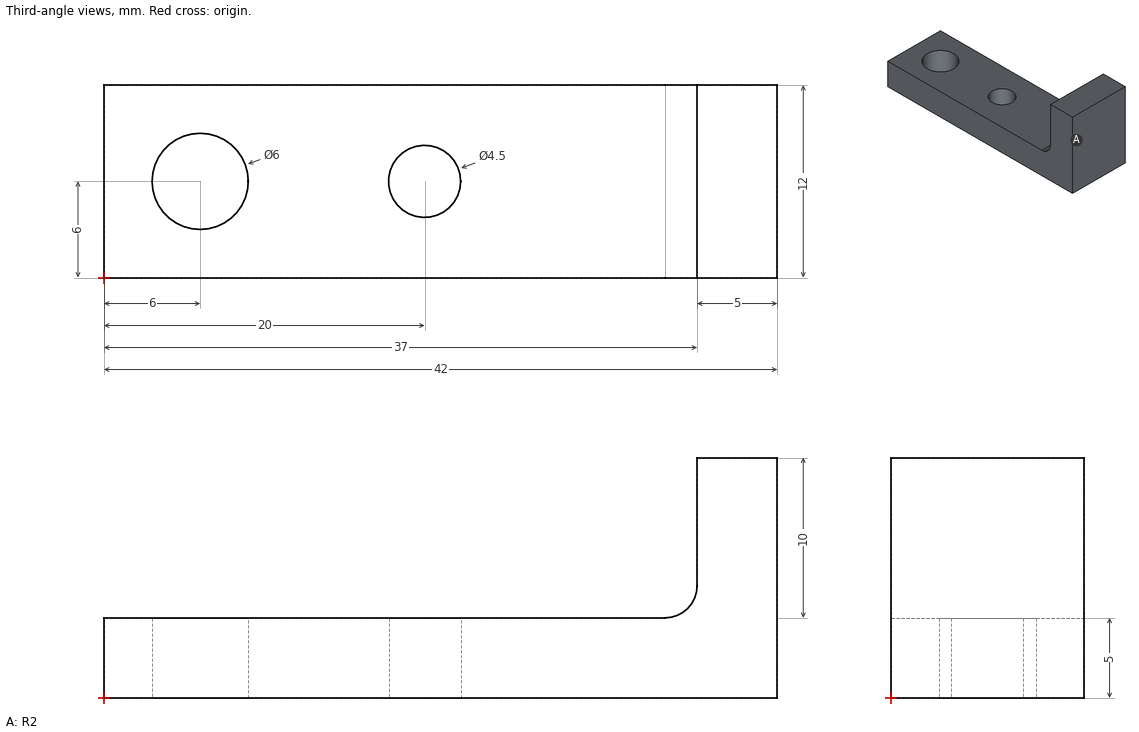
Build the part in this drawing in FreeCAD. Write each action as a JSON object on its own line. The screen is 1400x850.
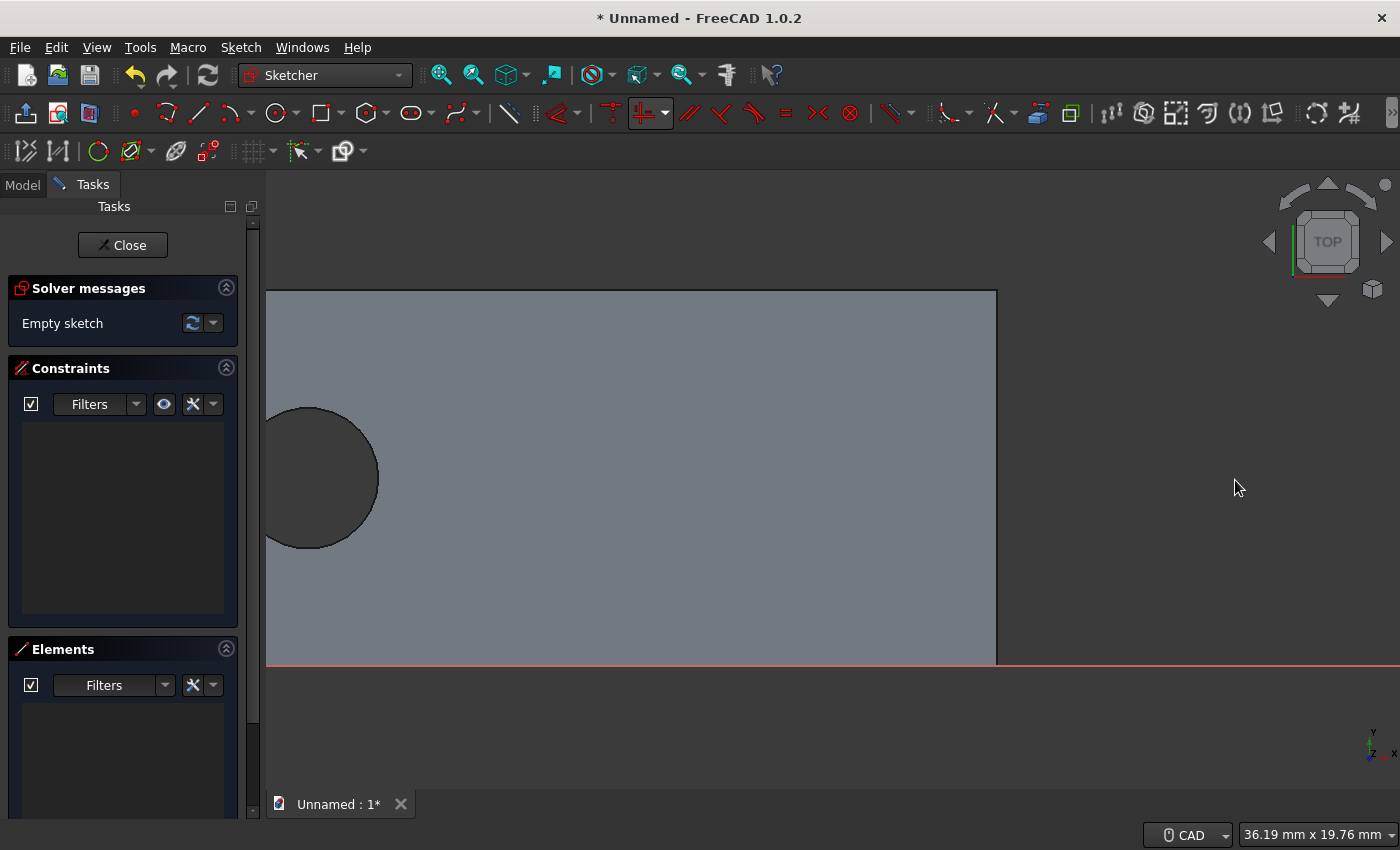
{"action": "key", "text": "g r"}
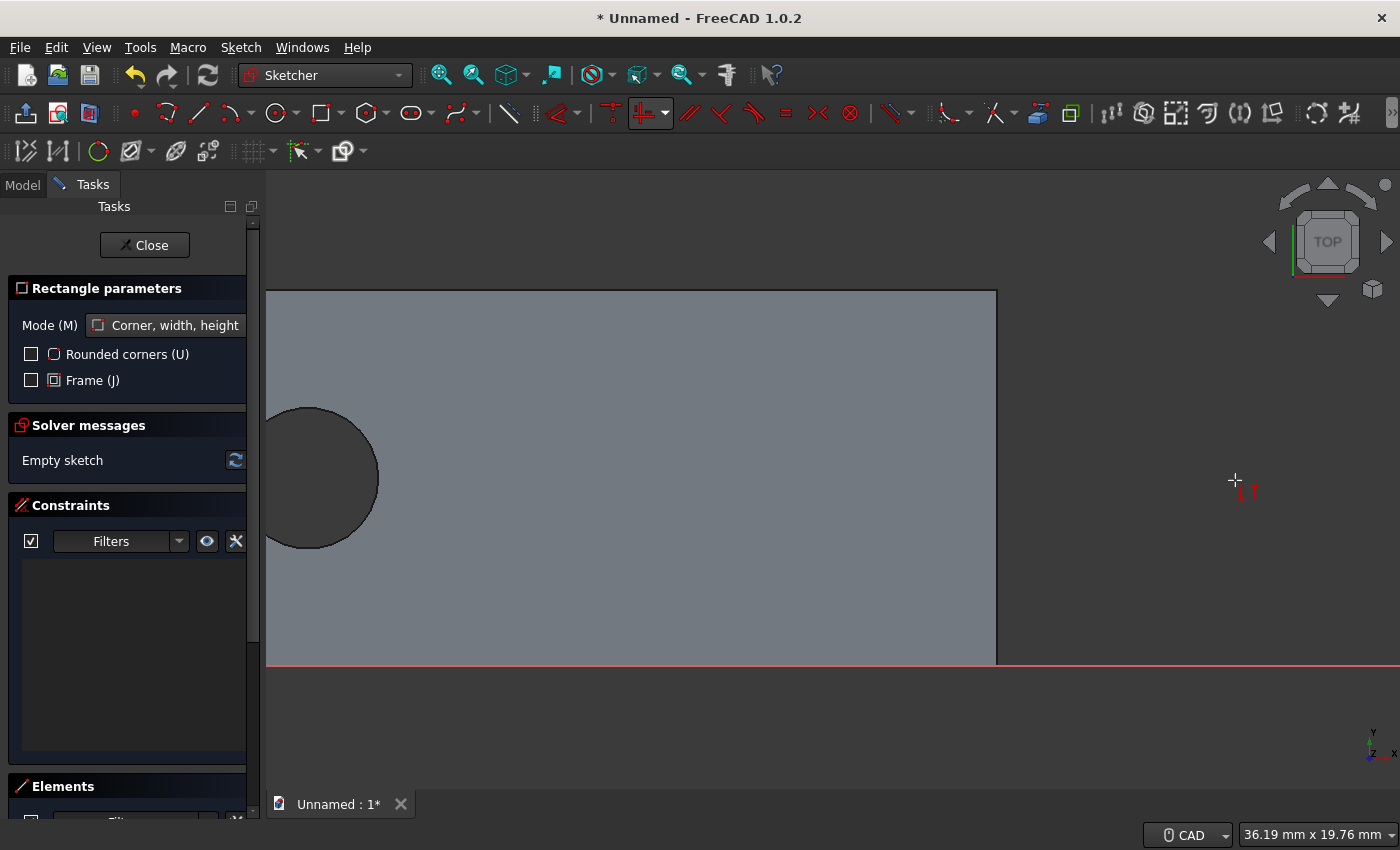
{"action": "left_click", "coordinate": [841, 290]}
{"action": "left_click", "coordinate": [997, 666]}
{"action": "key", "text": "Escape"}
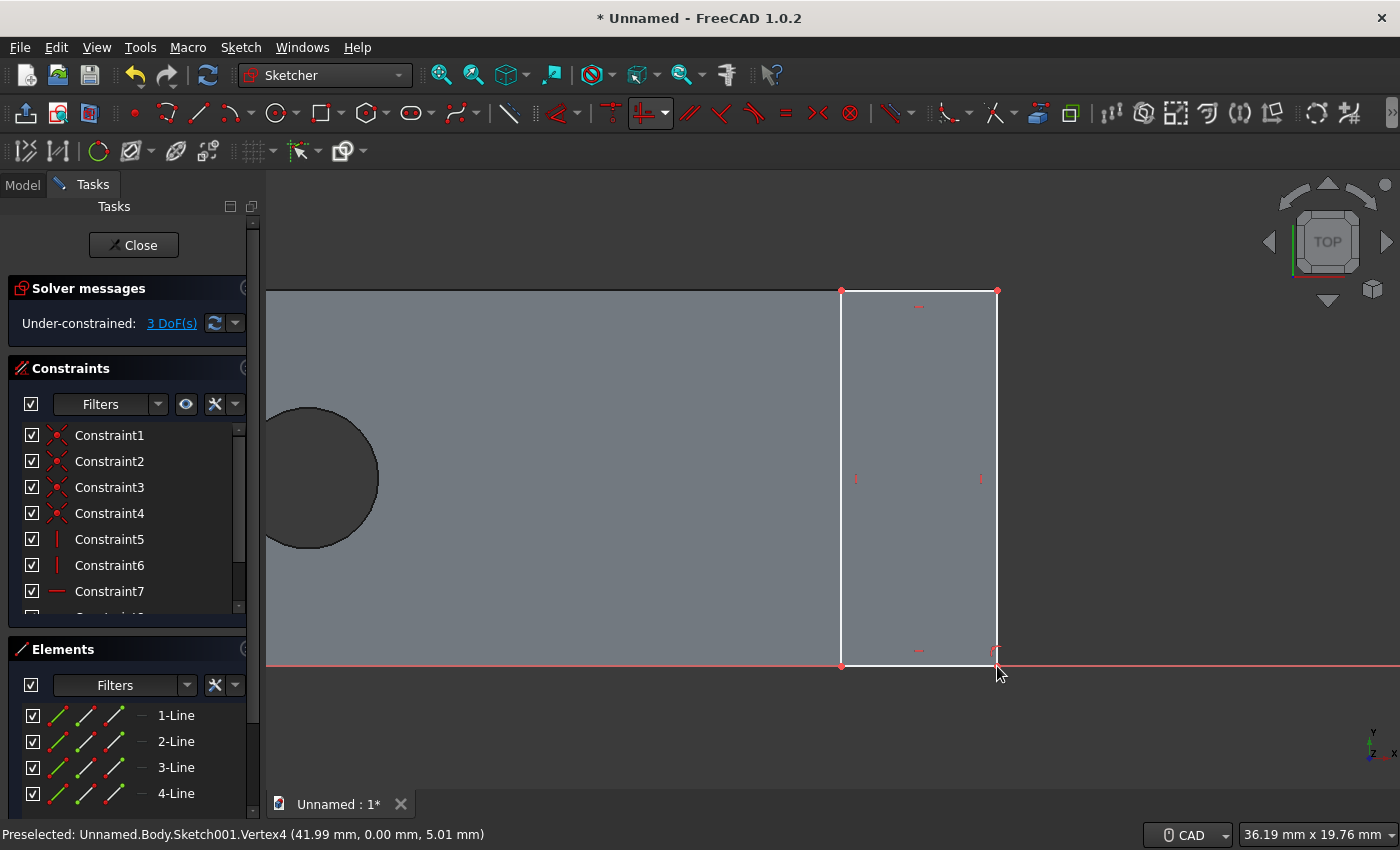
{"action": "left_click", "coordinate": [556, 114]}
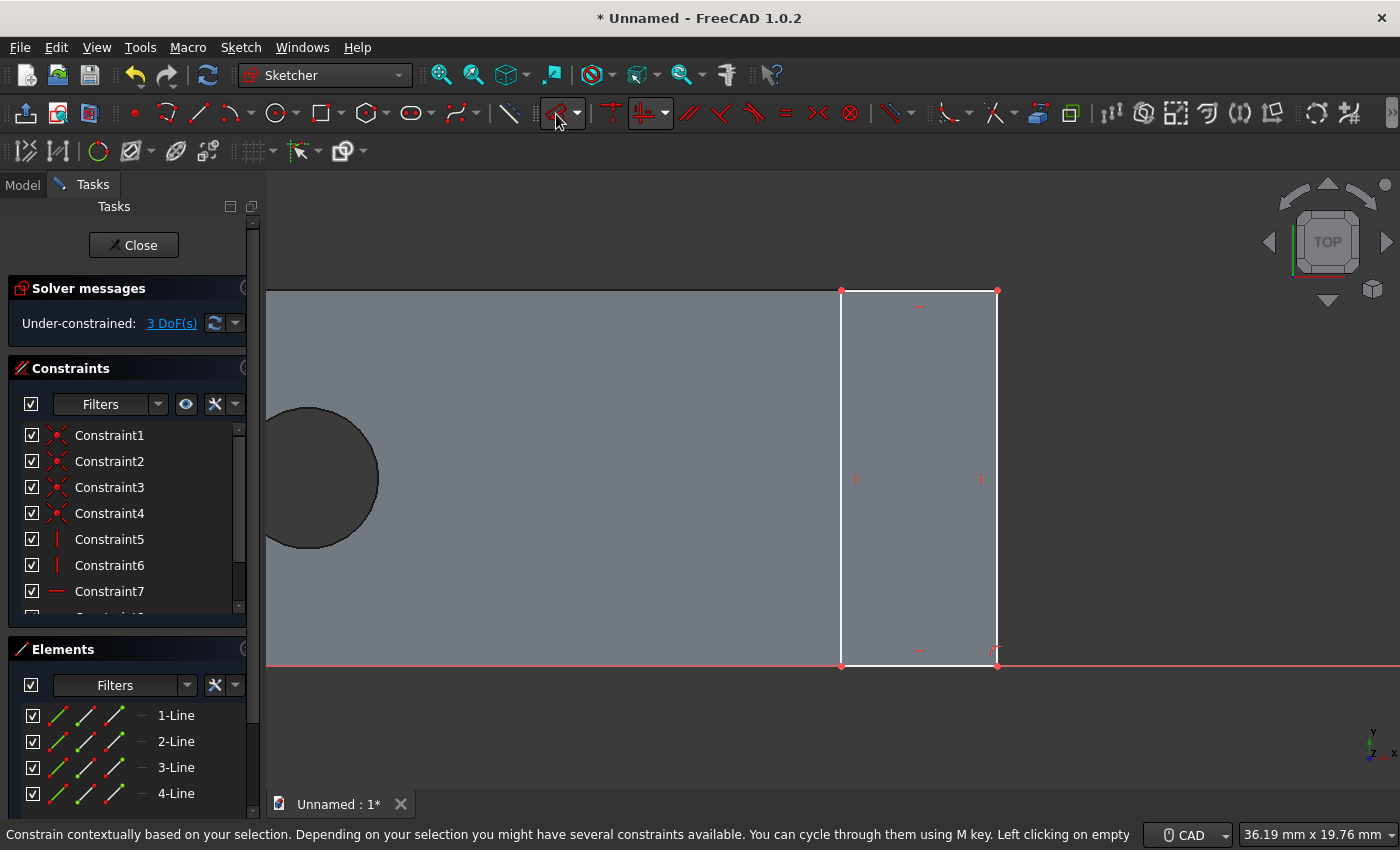
{"action": "left_click", "coordinate": [888, 666]}
{"action": "left_click", "coordinate": [919, 700]}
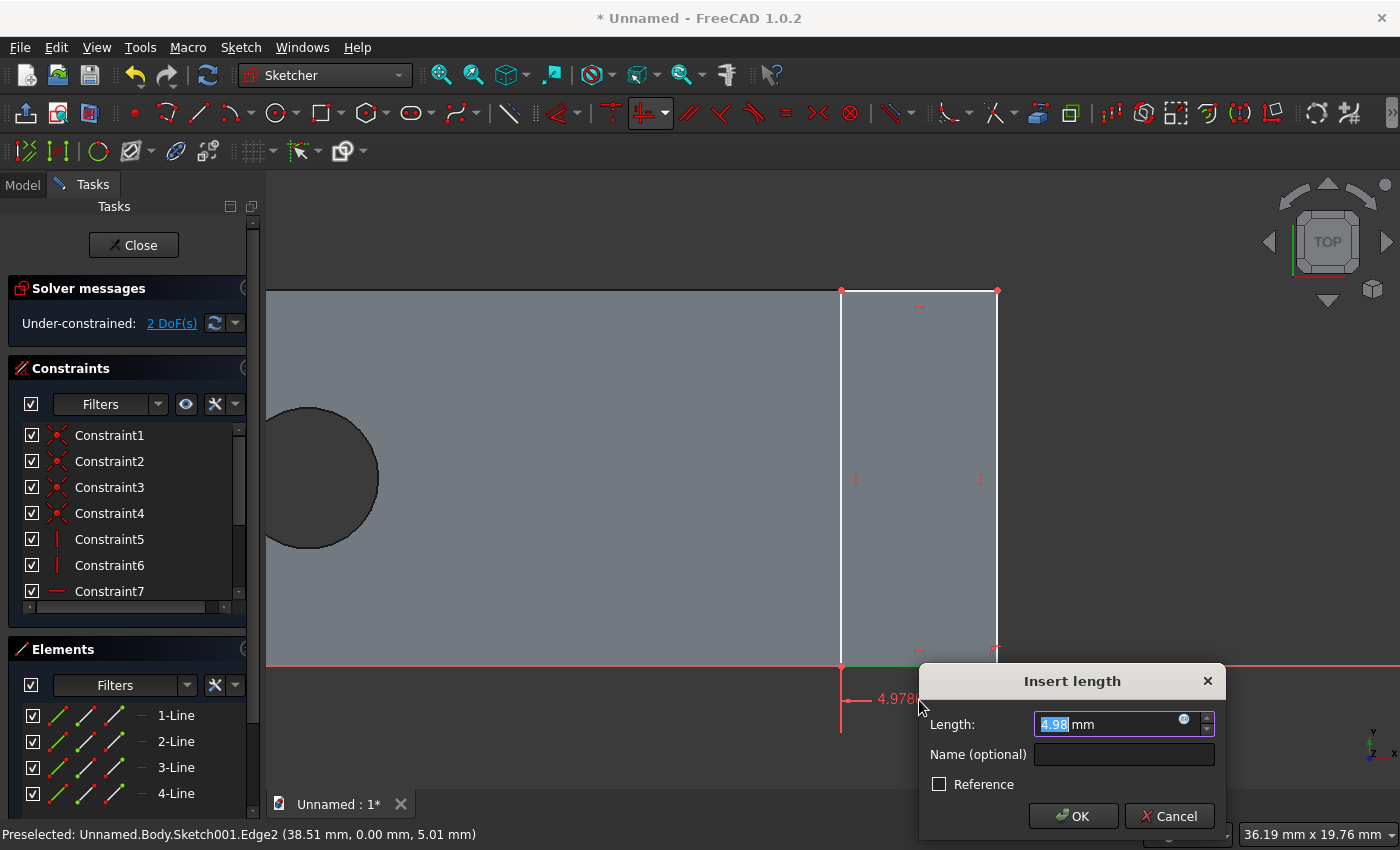
{"action": "type", "text": "5"}
{"action": "key", "text": "Return"}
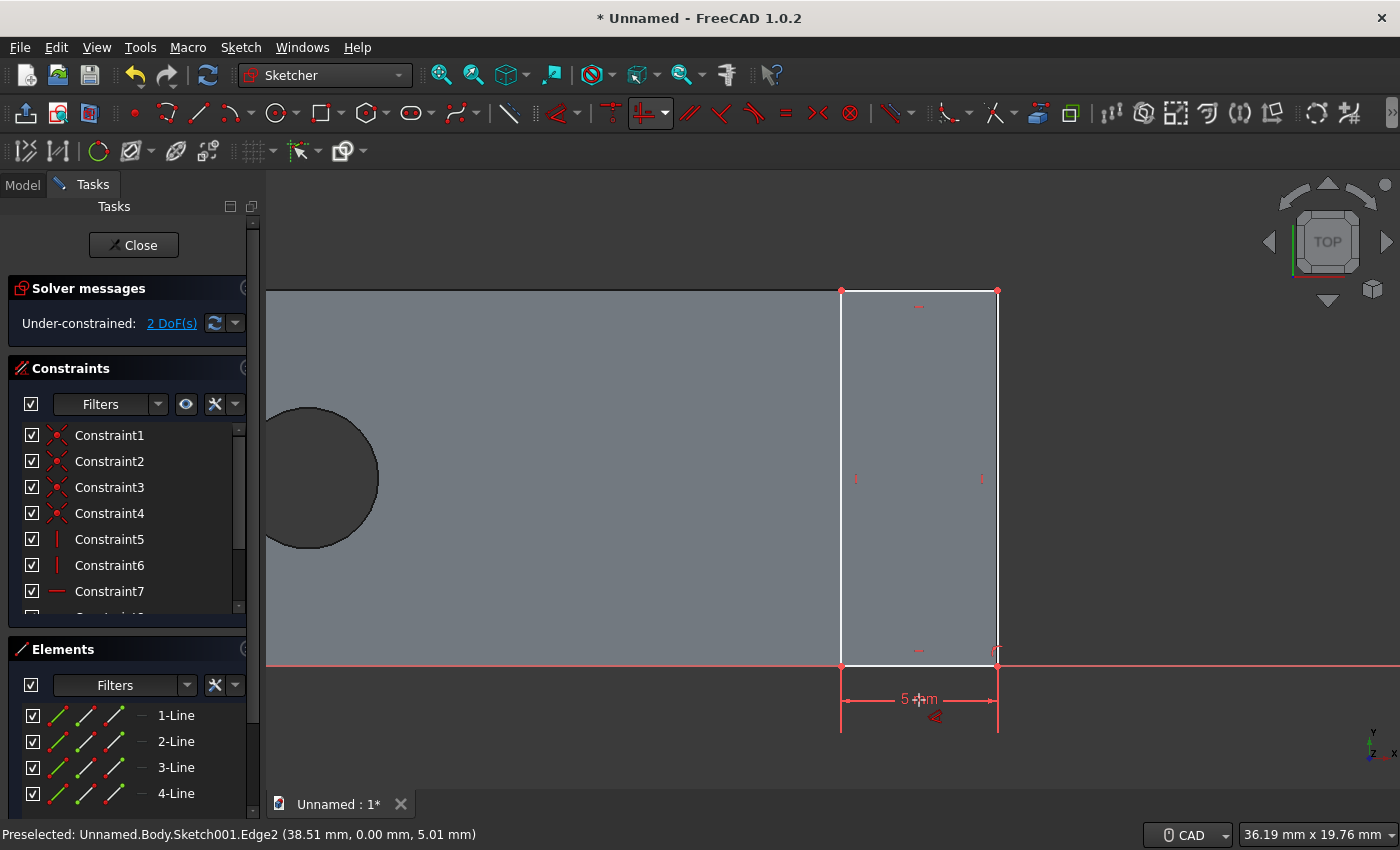
{"action": "left_click", "coordinate": [841, 404]}
{"action": "left_click", "coordinate": [807, 479]}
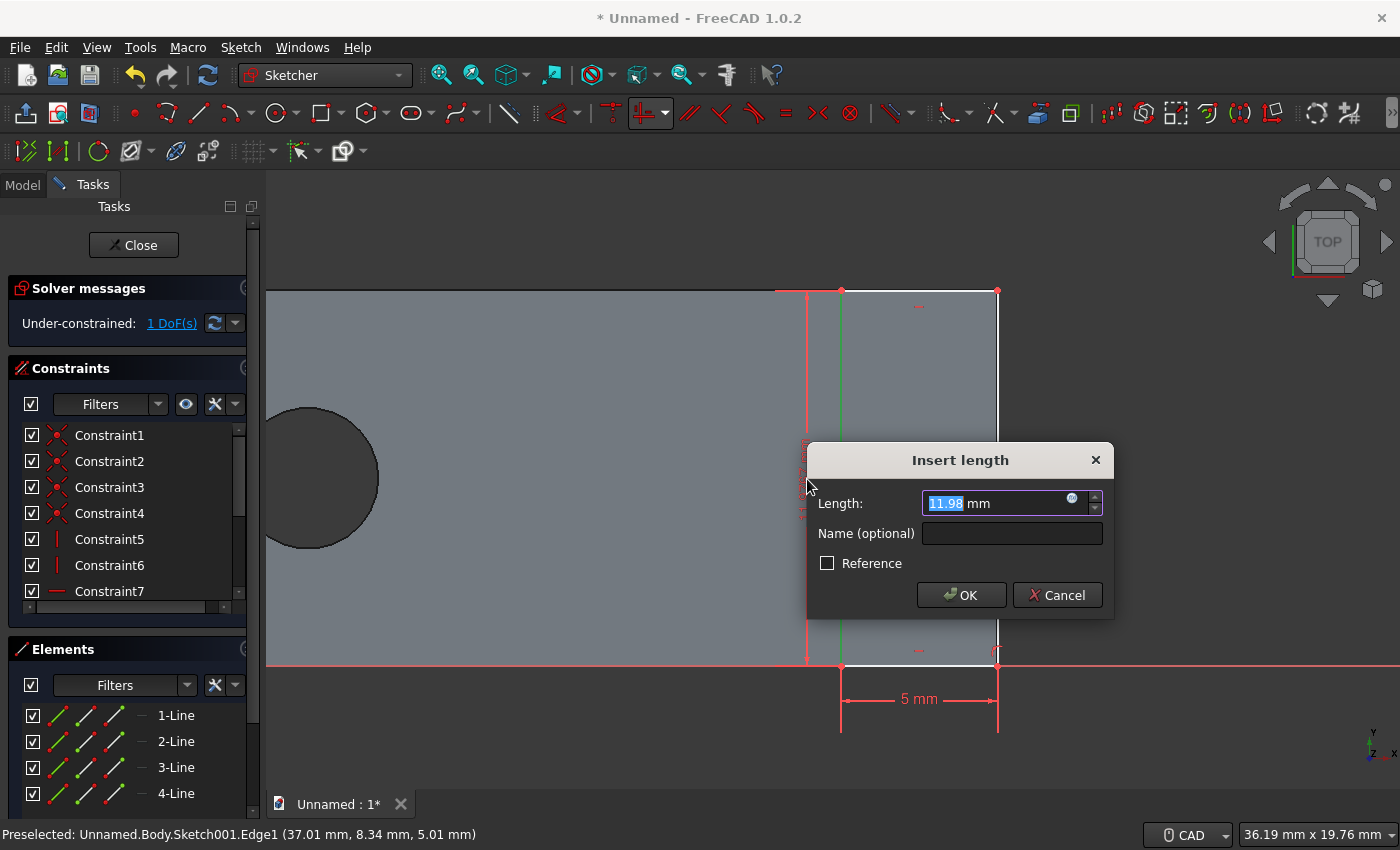
{"action": "type", "text": "12"}
{"action": "key", "text": "Return"}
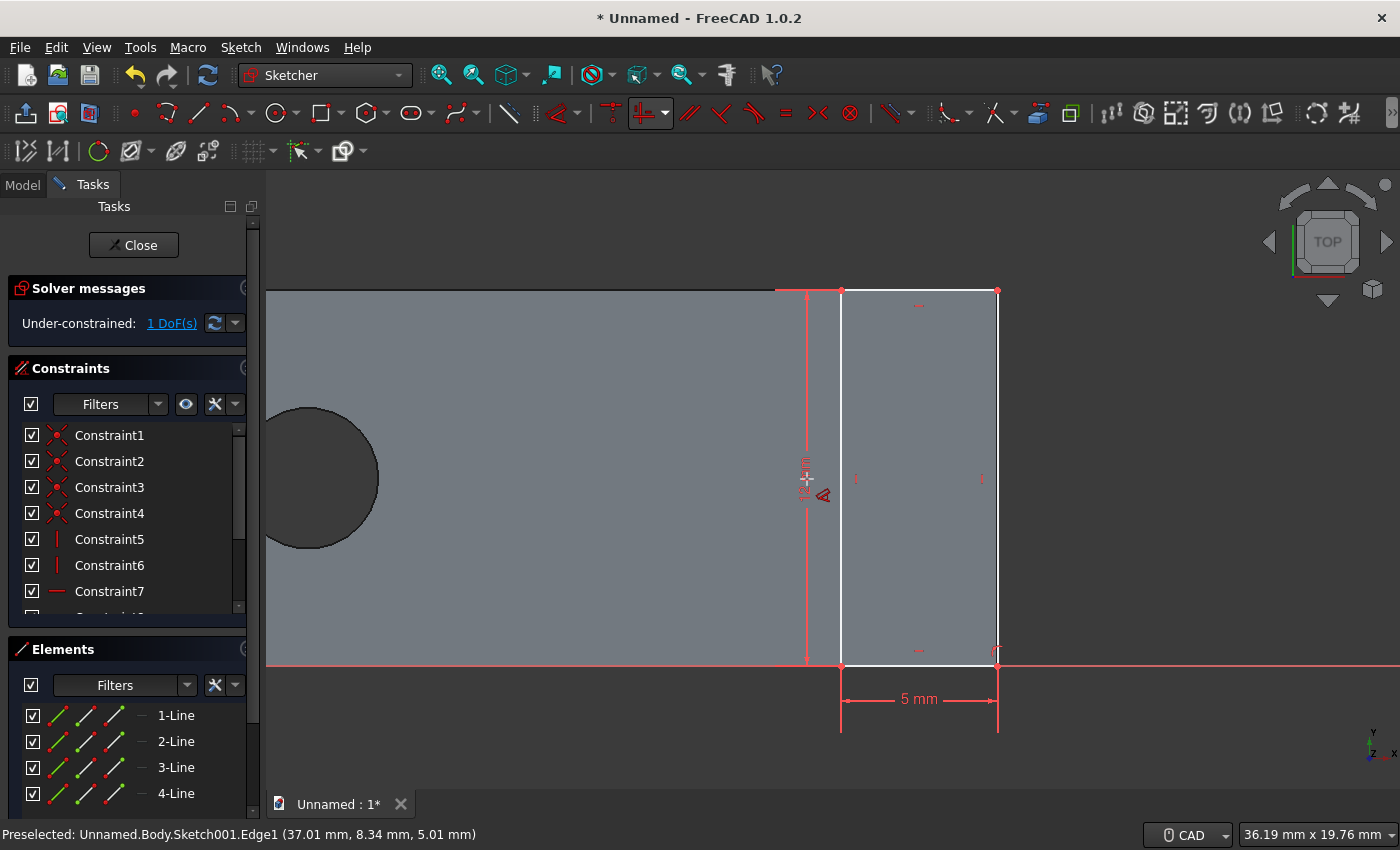
{"action": "left_click", "coordinate": [841, 290]}
{"action": "left_click", "coordinate": [568, 700]}